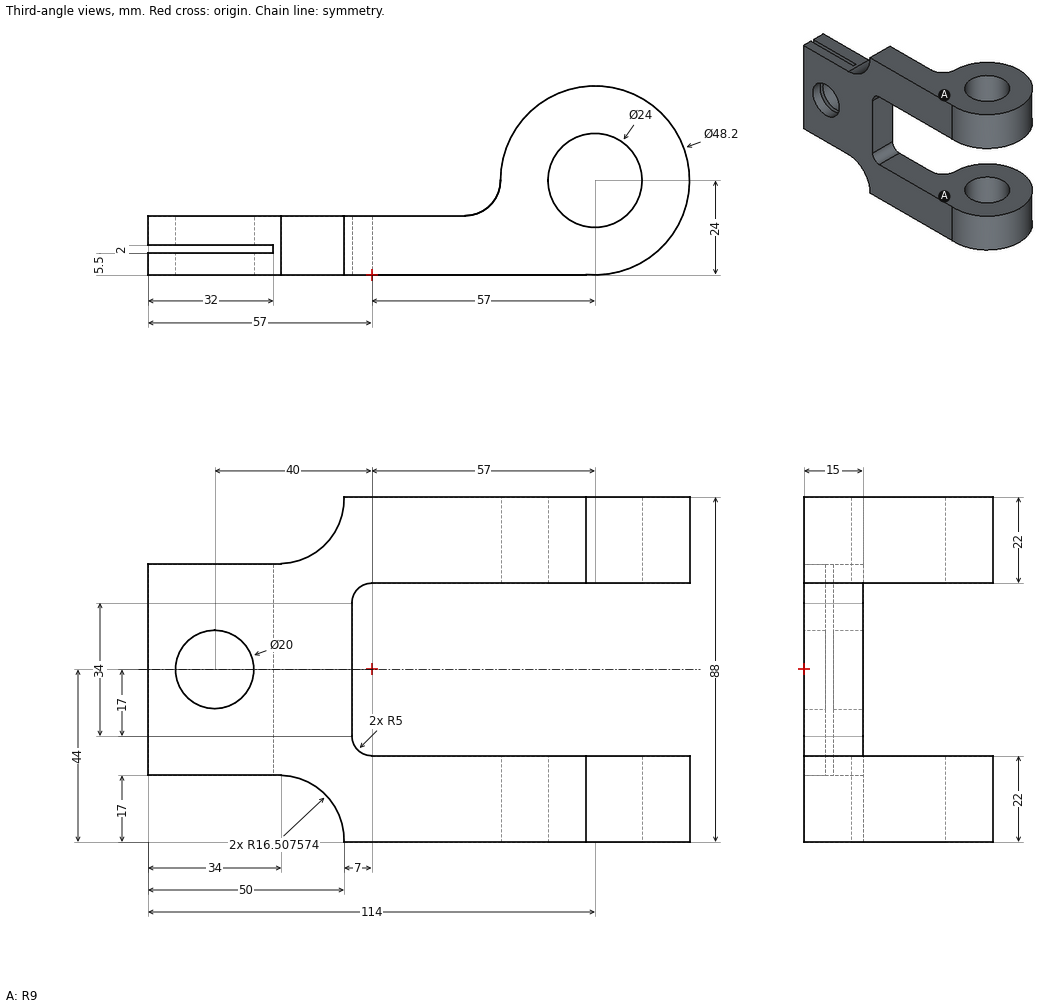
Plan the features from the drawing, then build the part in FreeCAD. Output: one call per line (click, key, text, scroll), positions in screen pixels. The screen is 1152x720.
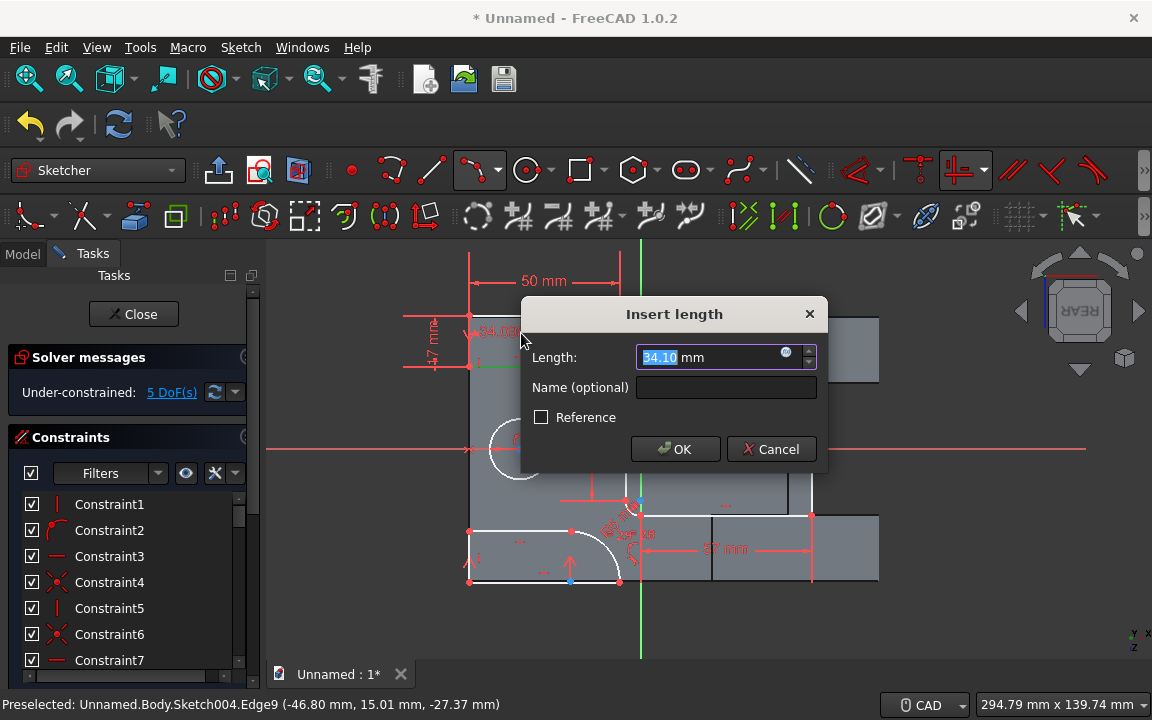
text(34)
key(Return)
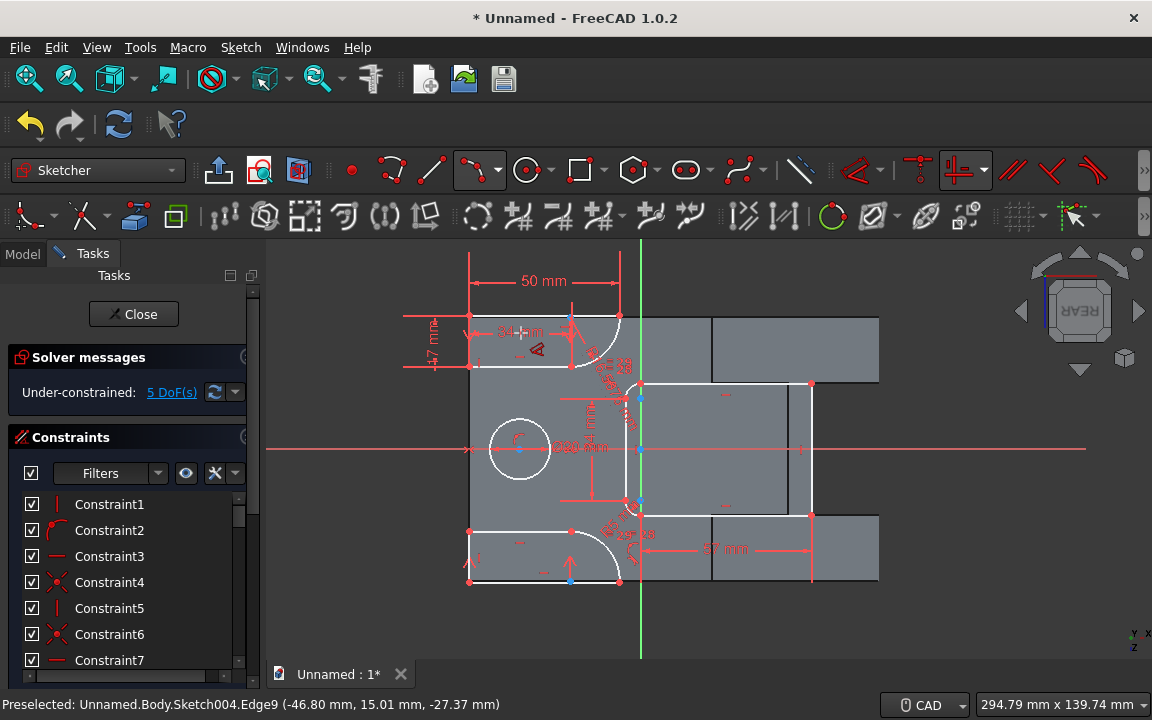
click(541, 532)
click(521, 566)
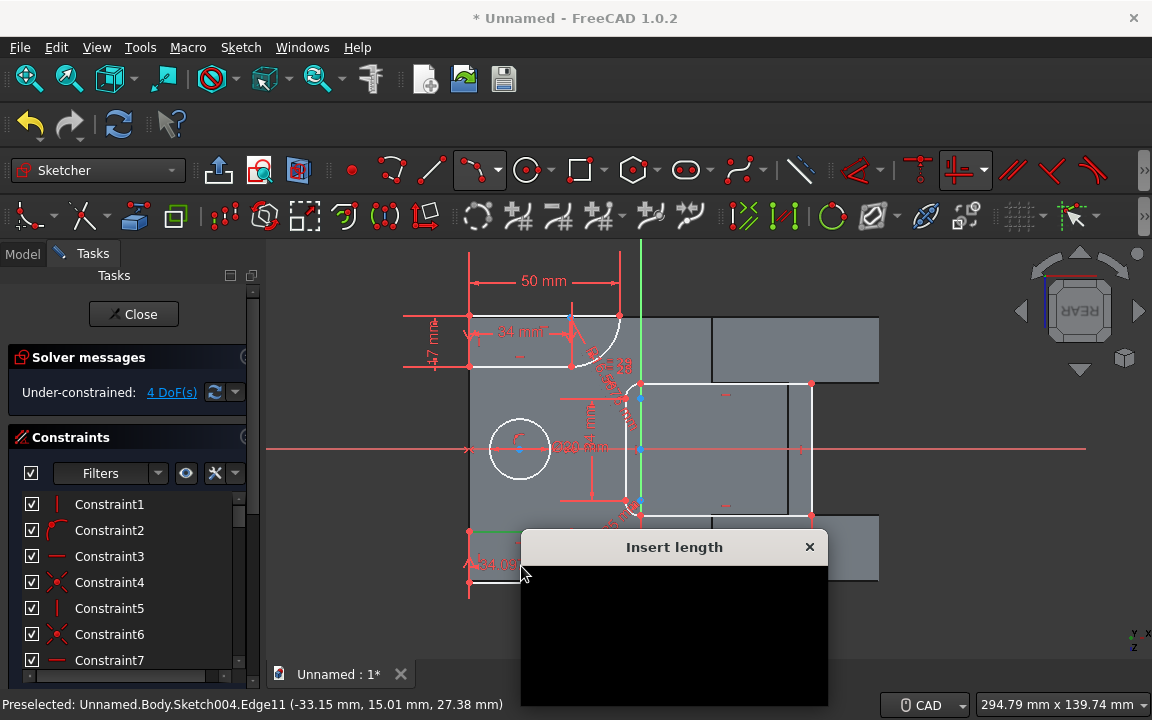
text(34)
key(Return)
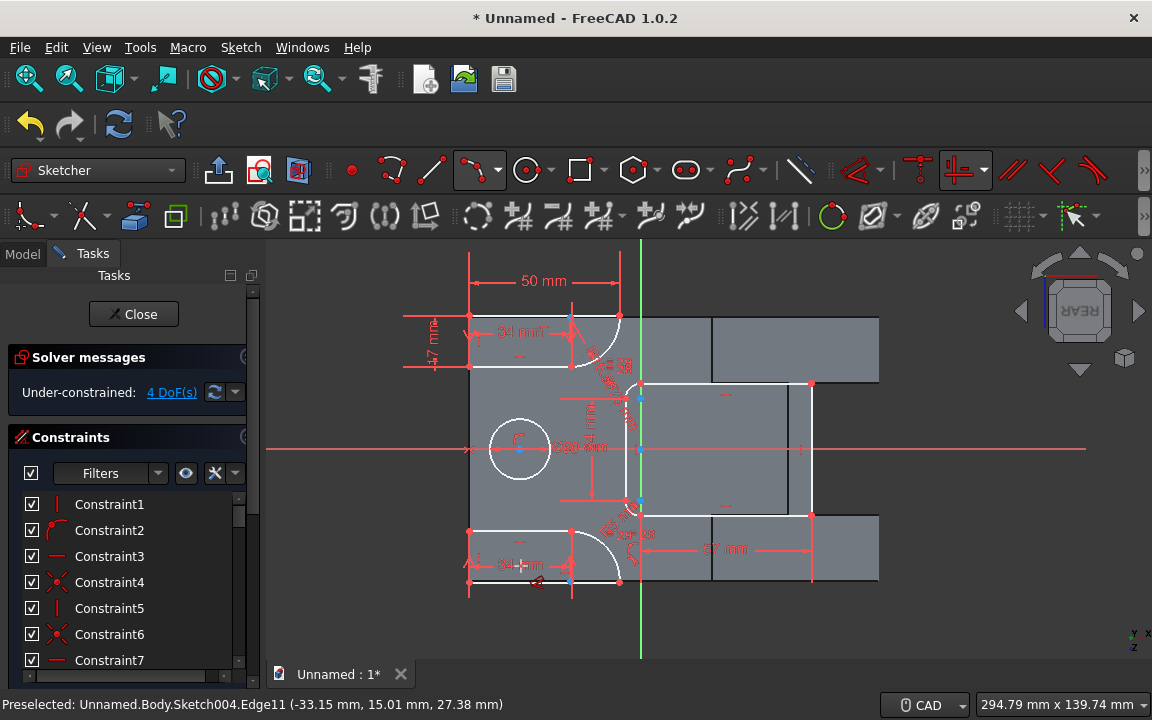
scroll(620, 316, up, 4)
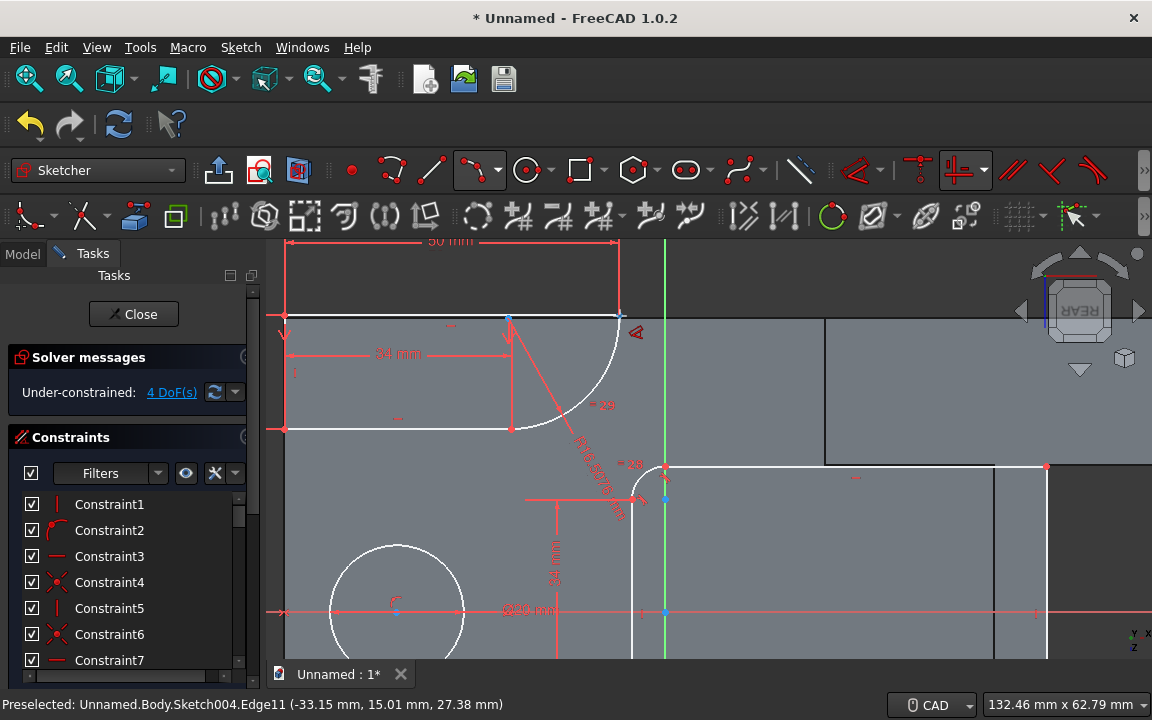
click(619, 315)
click(642, 281)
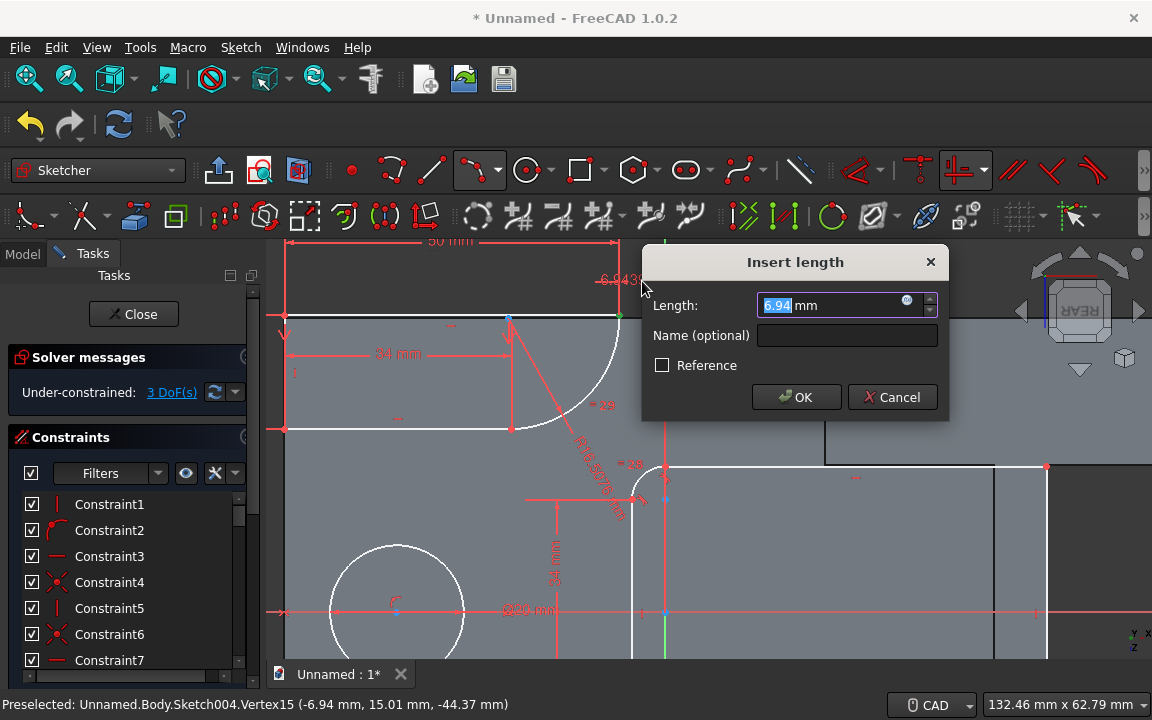
text(7)
key(Return)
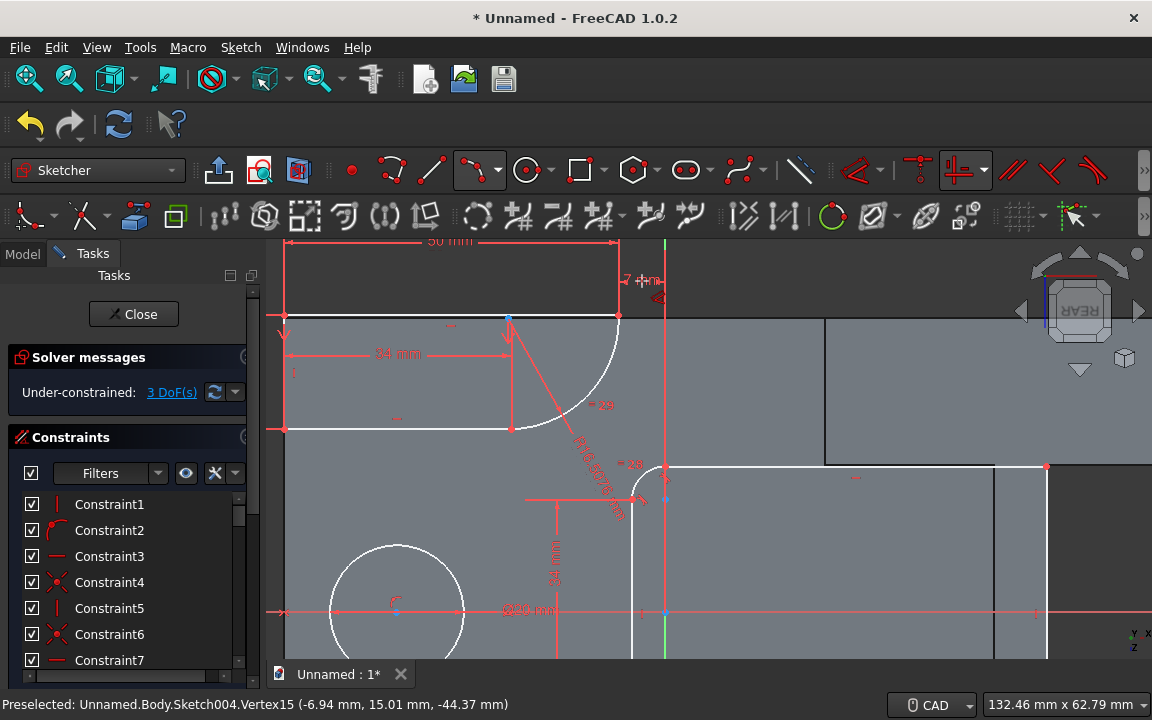
click(397, 612)
click(469, 578)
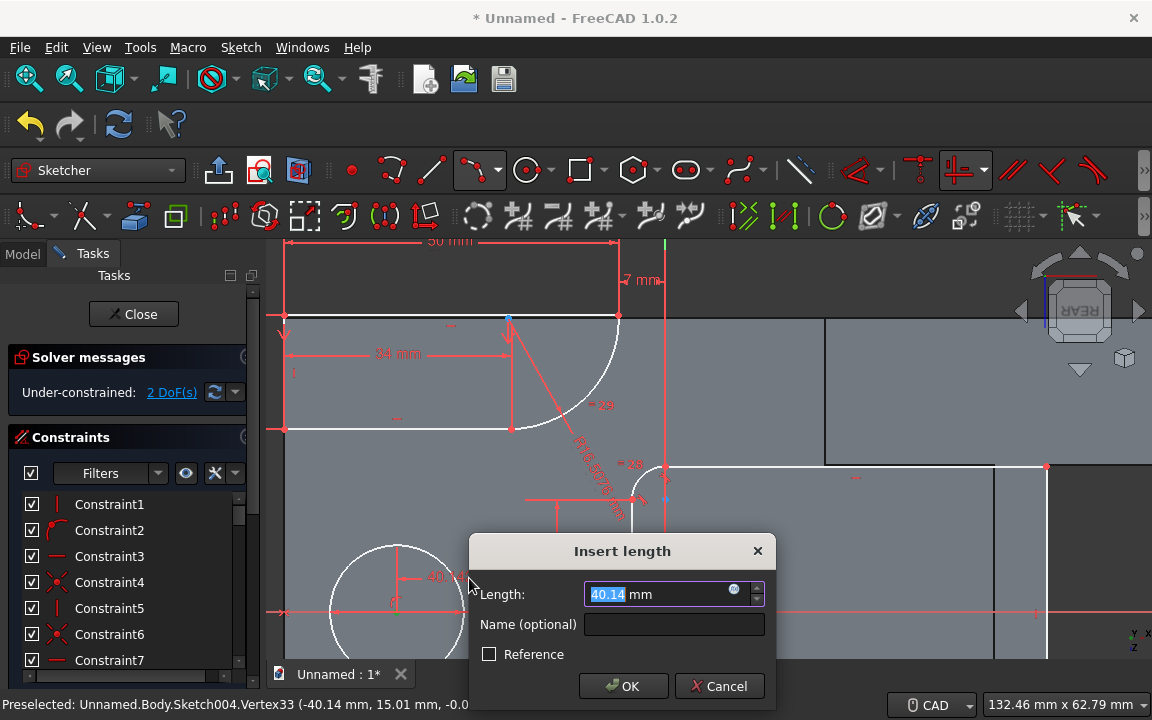
text(40)
key(Return)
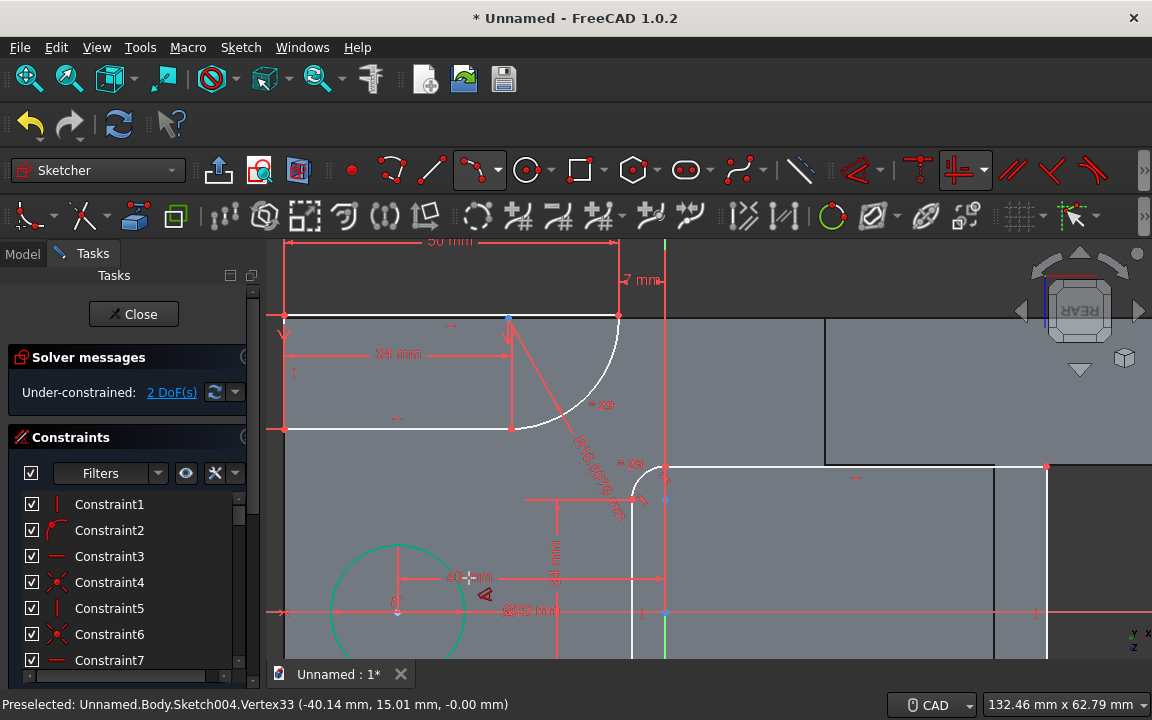
click(632, 500)
click(598, 530)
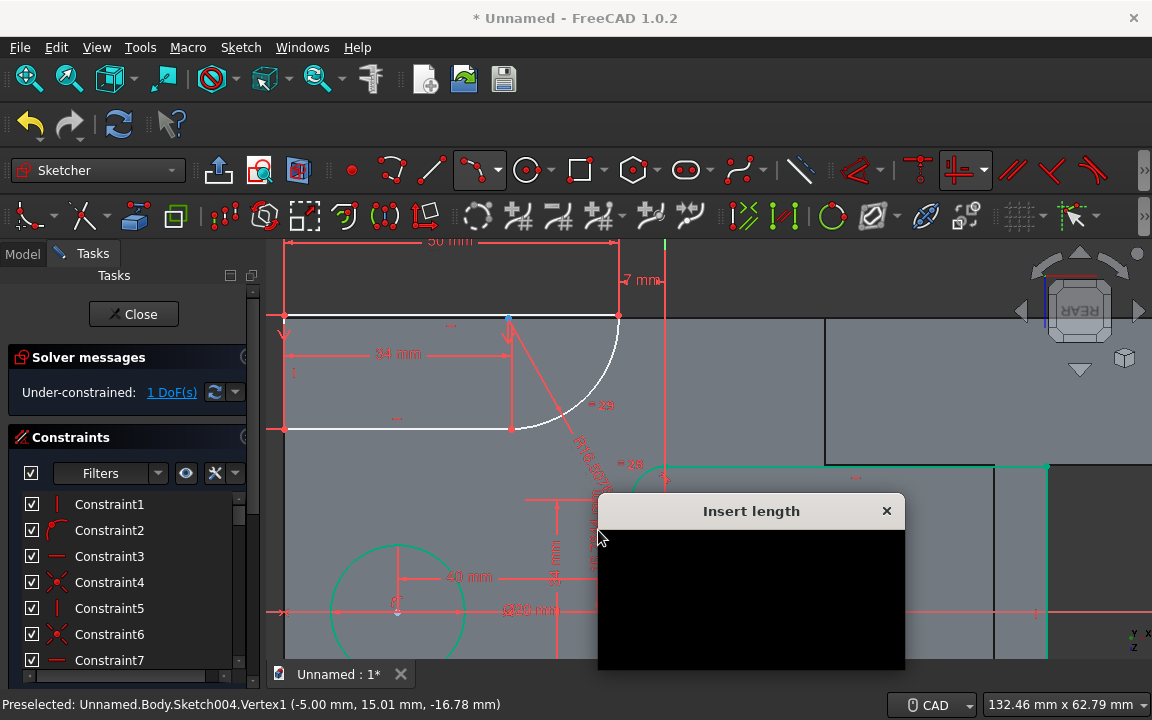
text(17)
key(Return)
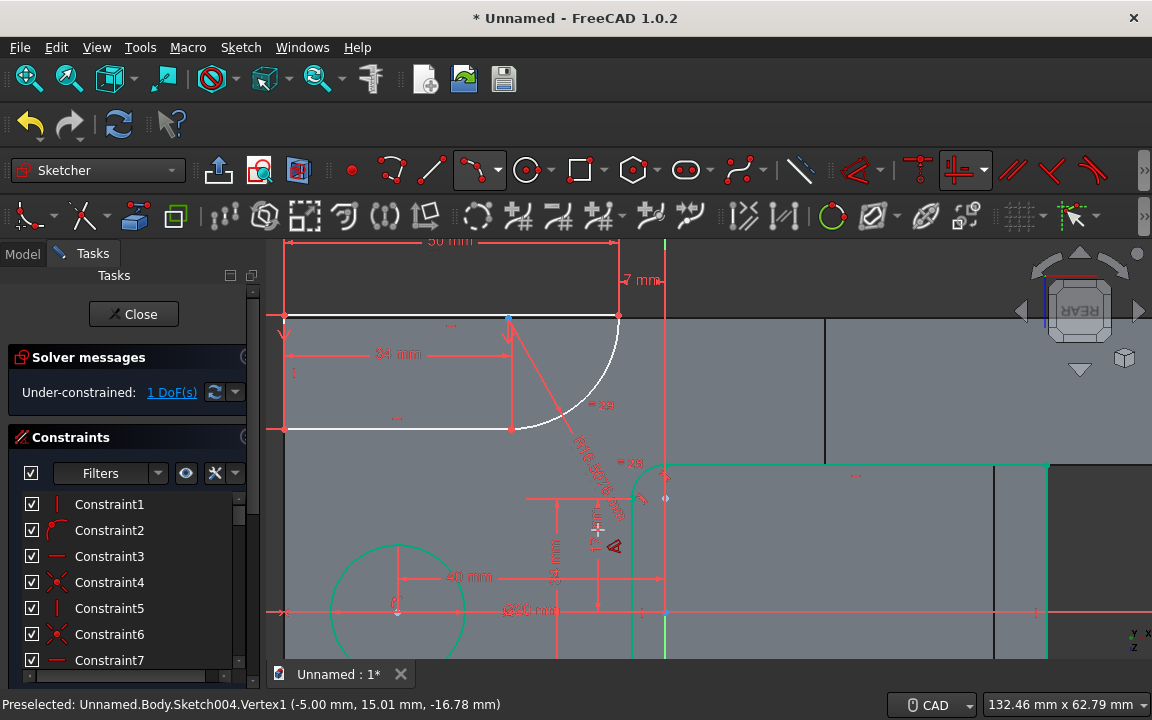
click(619, 315)
click(585, 360)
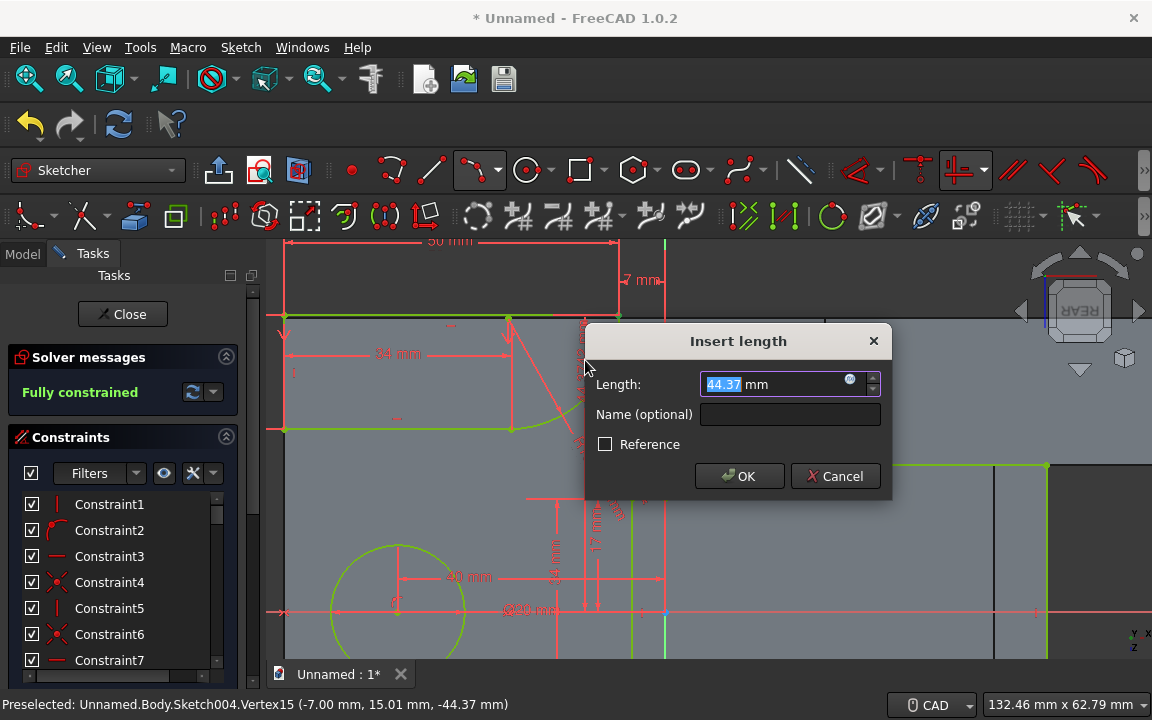
text(44)
key(Return)
key(Escape)